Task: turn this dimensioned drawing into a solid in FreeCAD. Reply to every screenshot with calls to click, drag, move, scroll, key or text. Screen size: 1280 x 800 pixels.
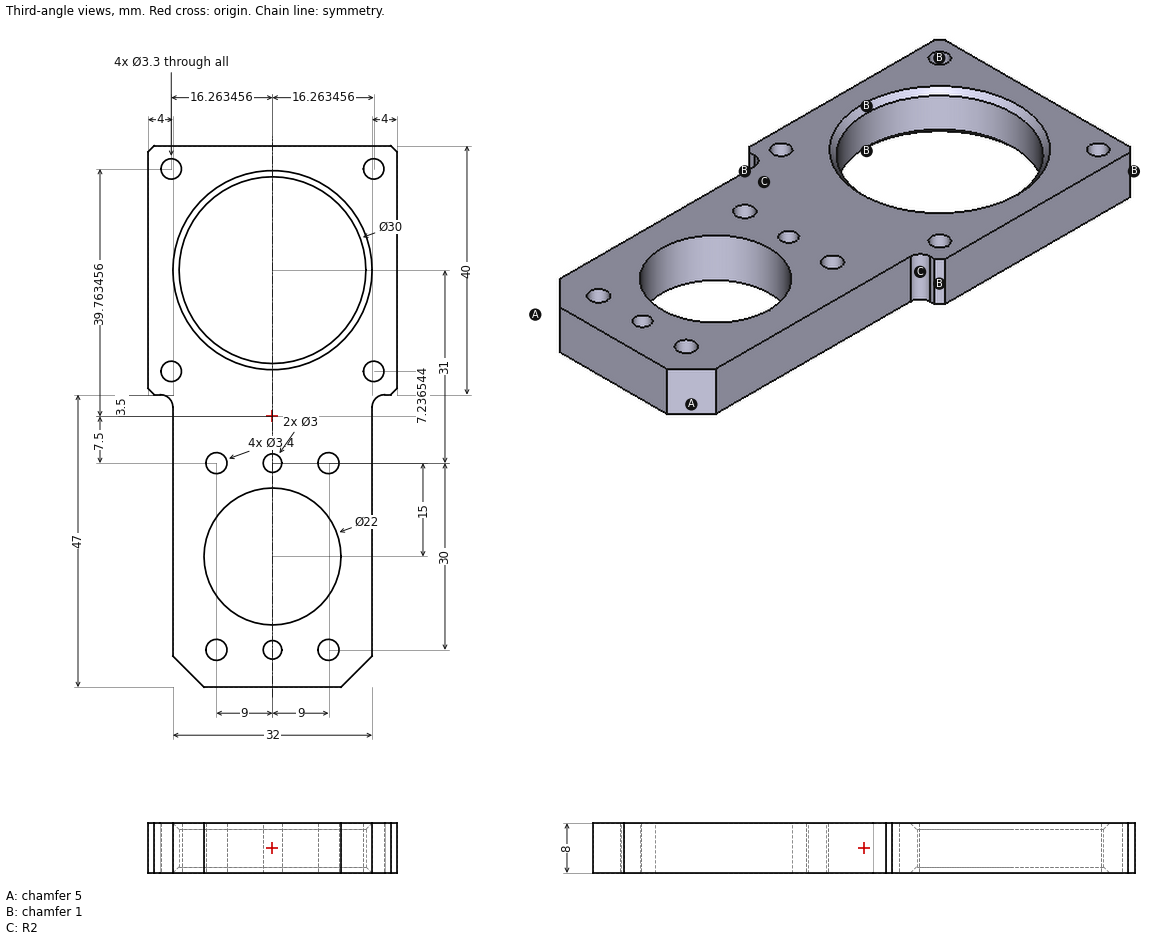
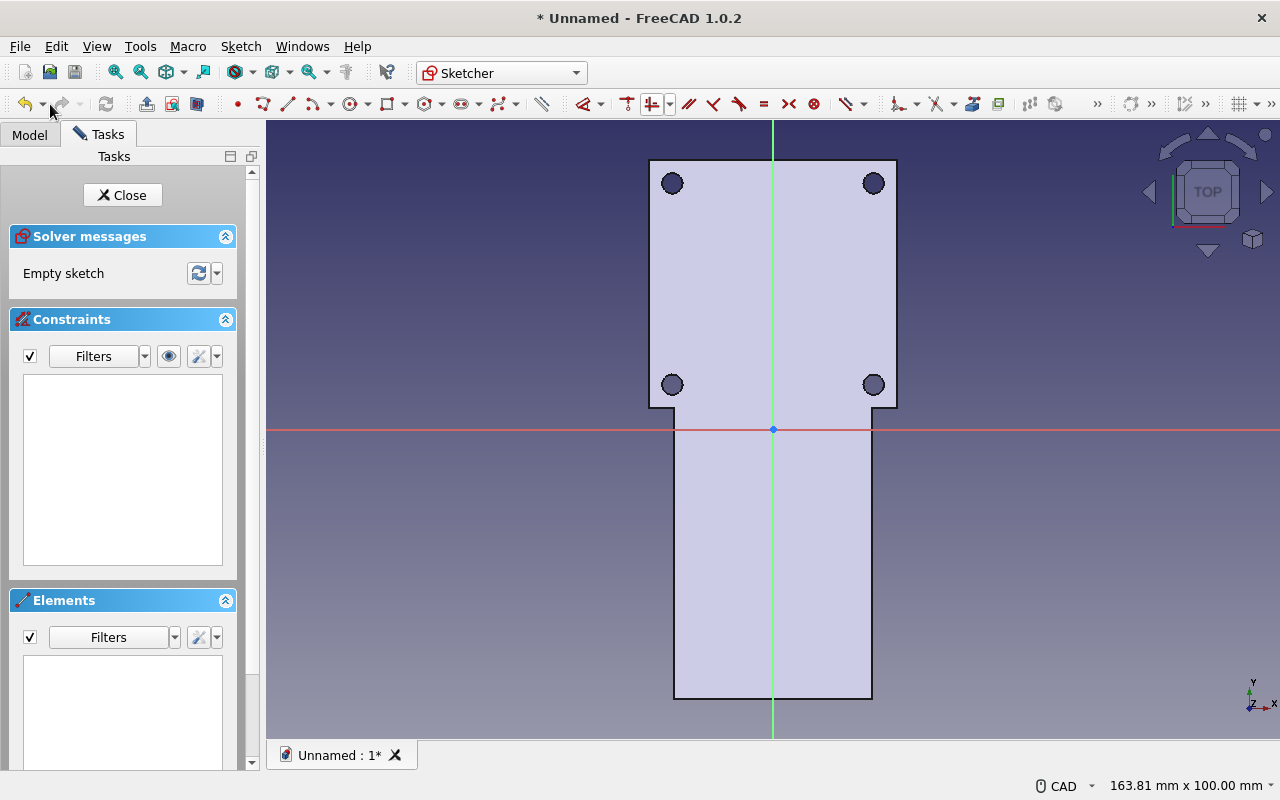
scroll(912, 711, up, 2)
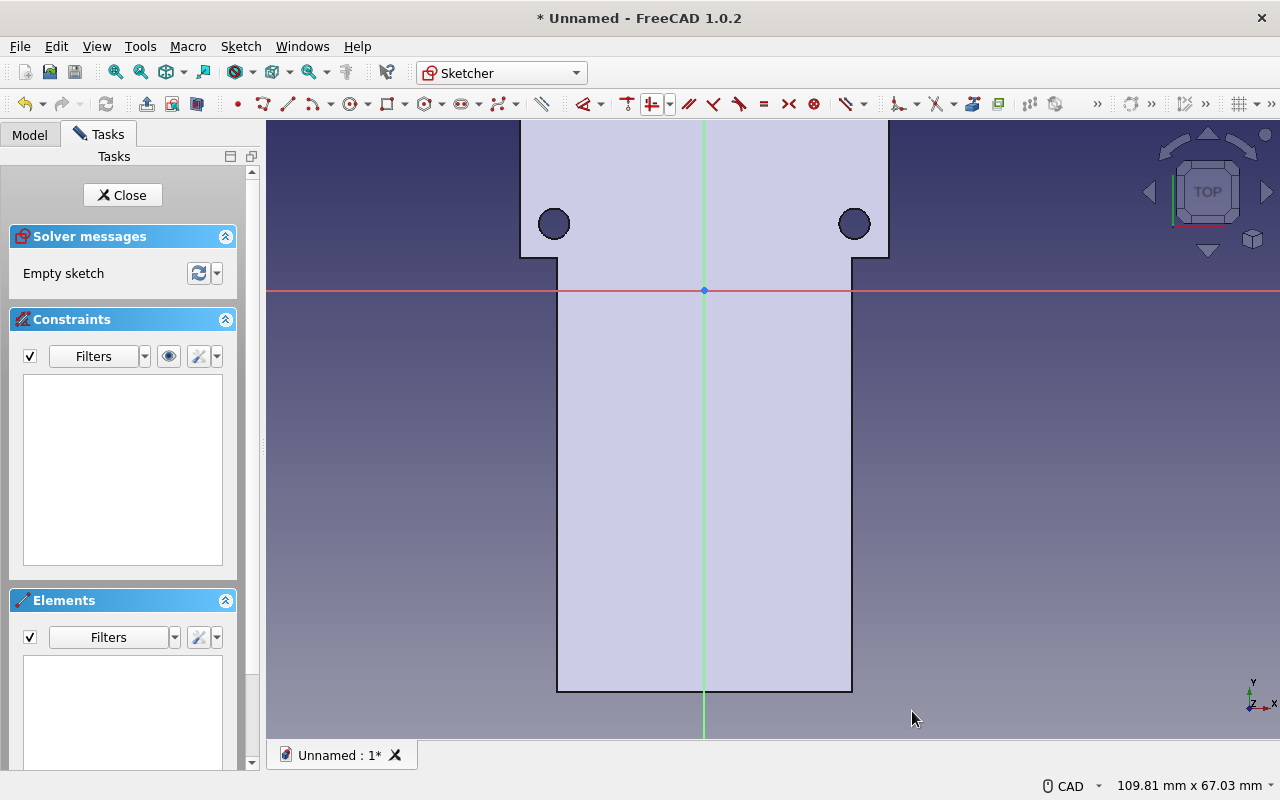
click(350, 104)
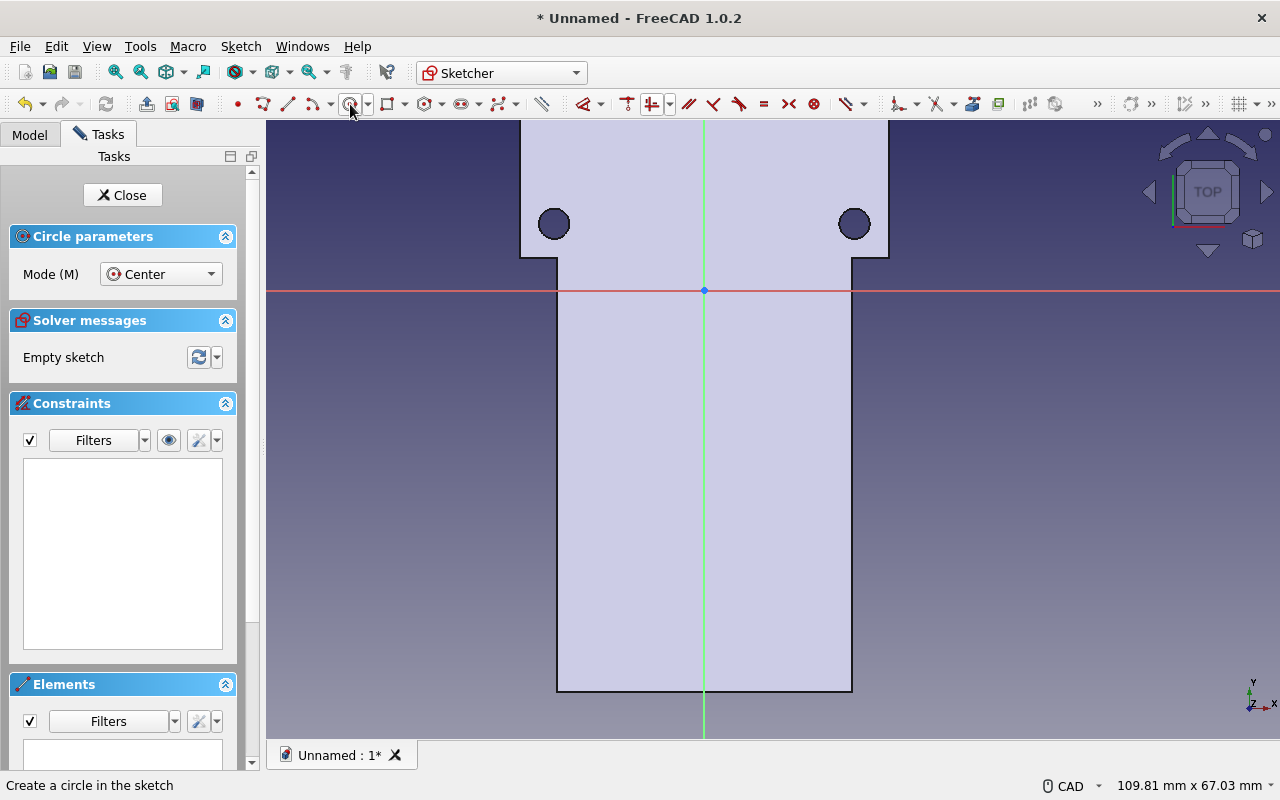
scroll(621, 360, up, 2)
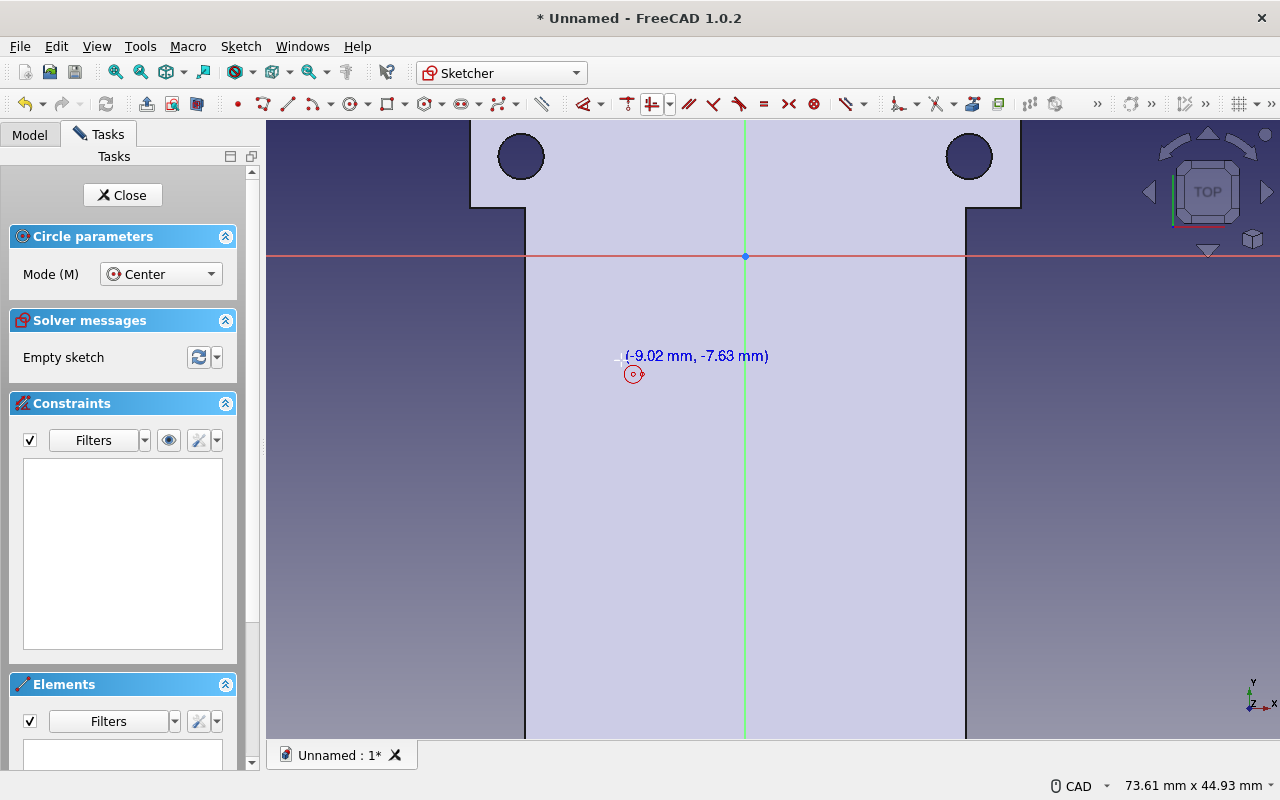
click(621, 360)
click(638, 343)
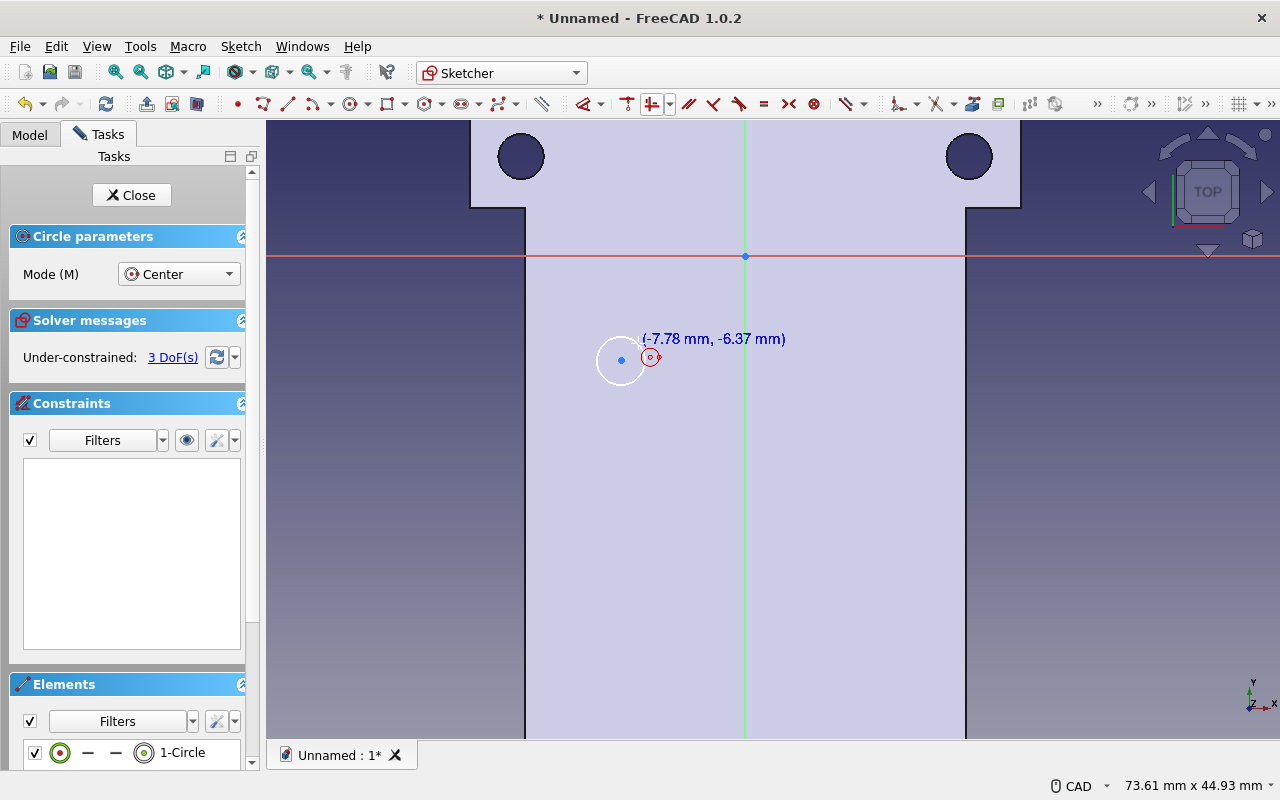
click(869, 360)
click(886, 343)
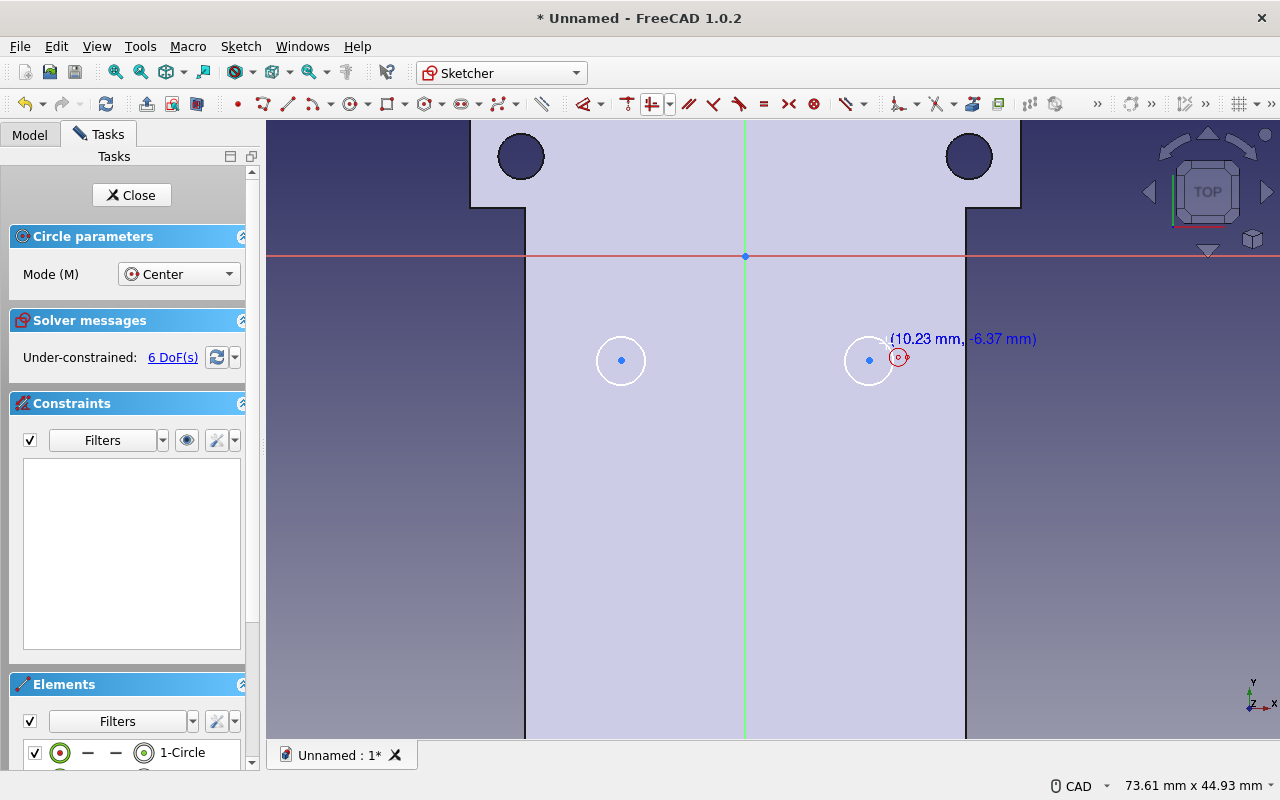
scroll(622, 233, down, 2)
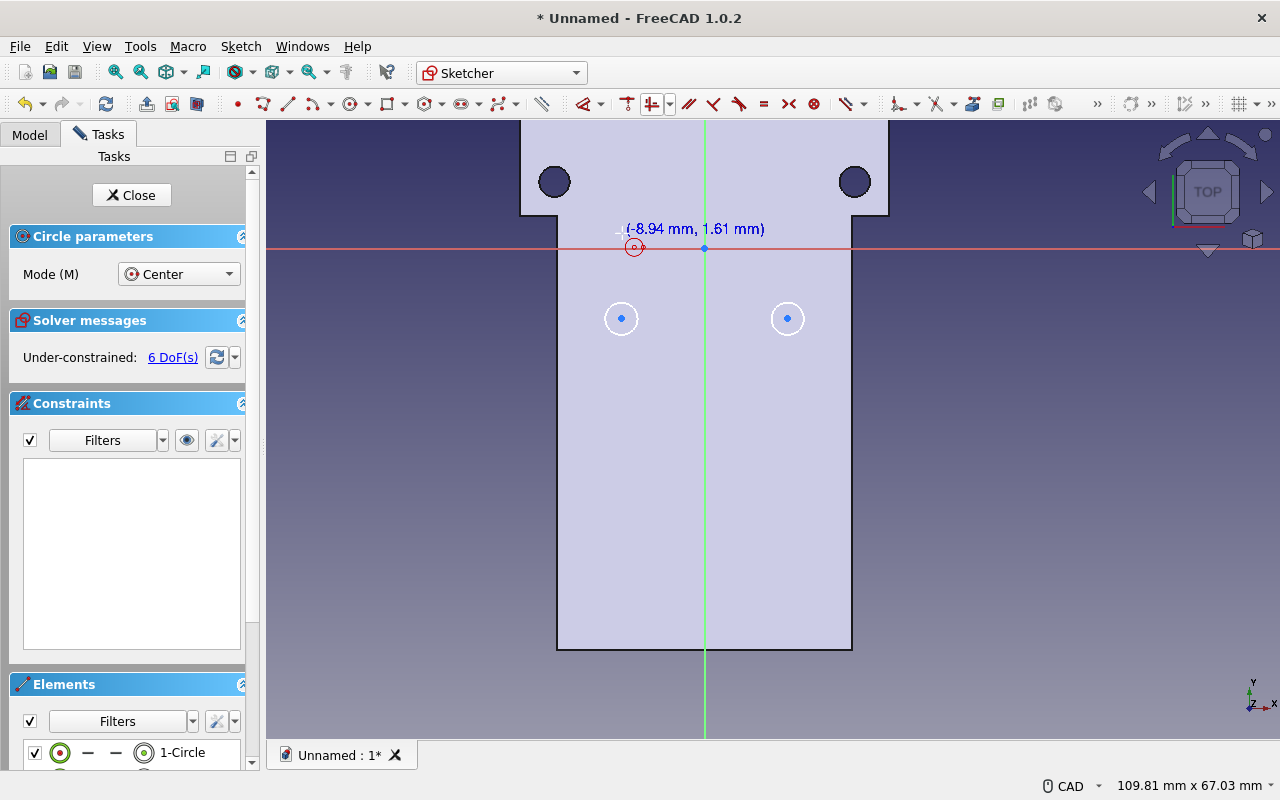
scroll(788, 595, up, 2)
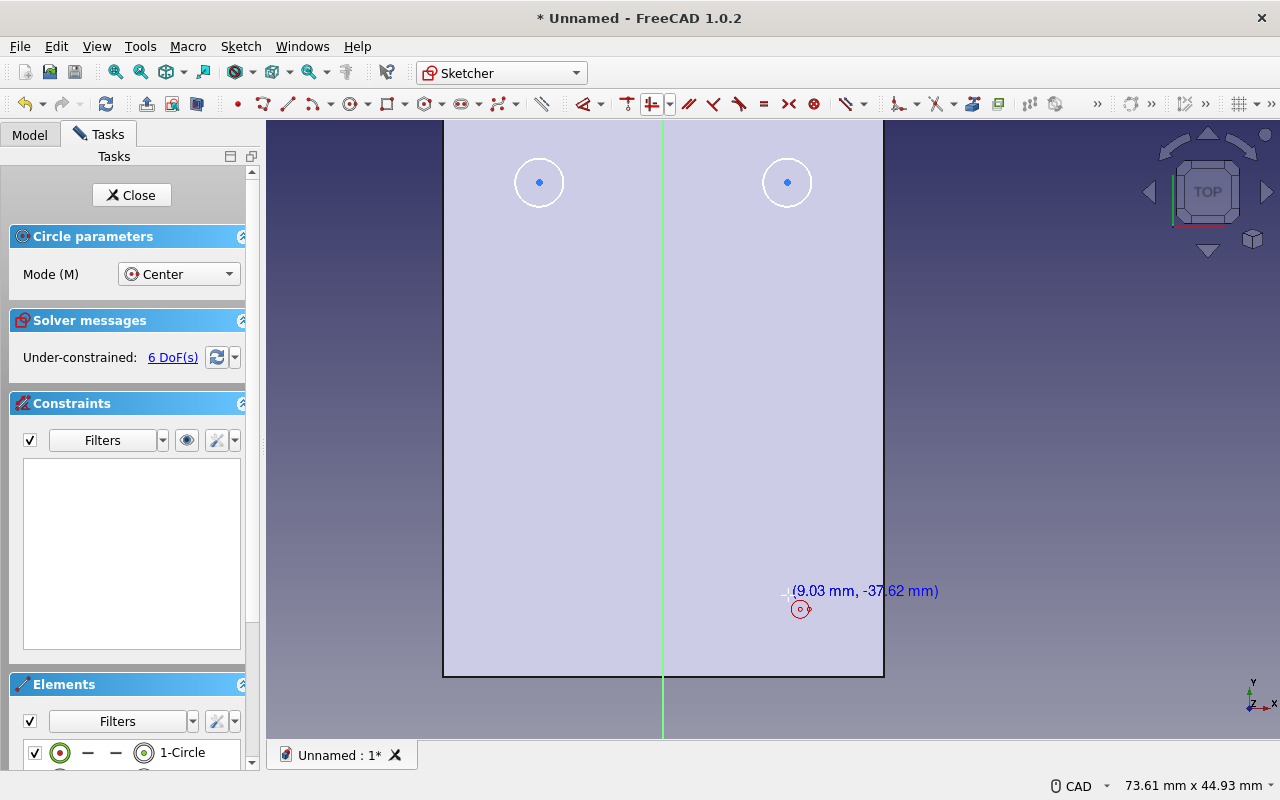
click(787, 595)
click(804, 578)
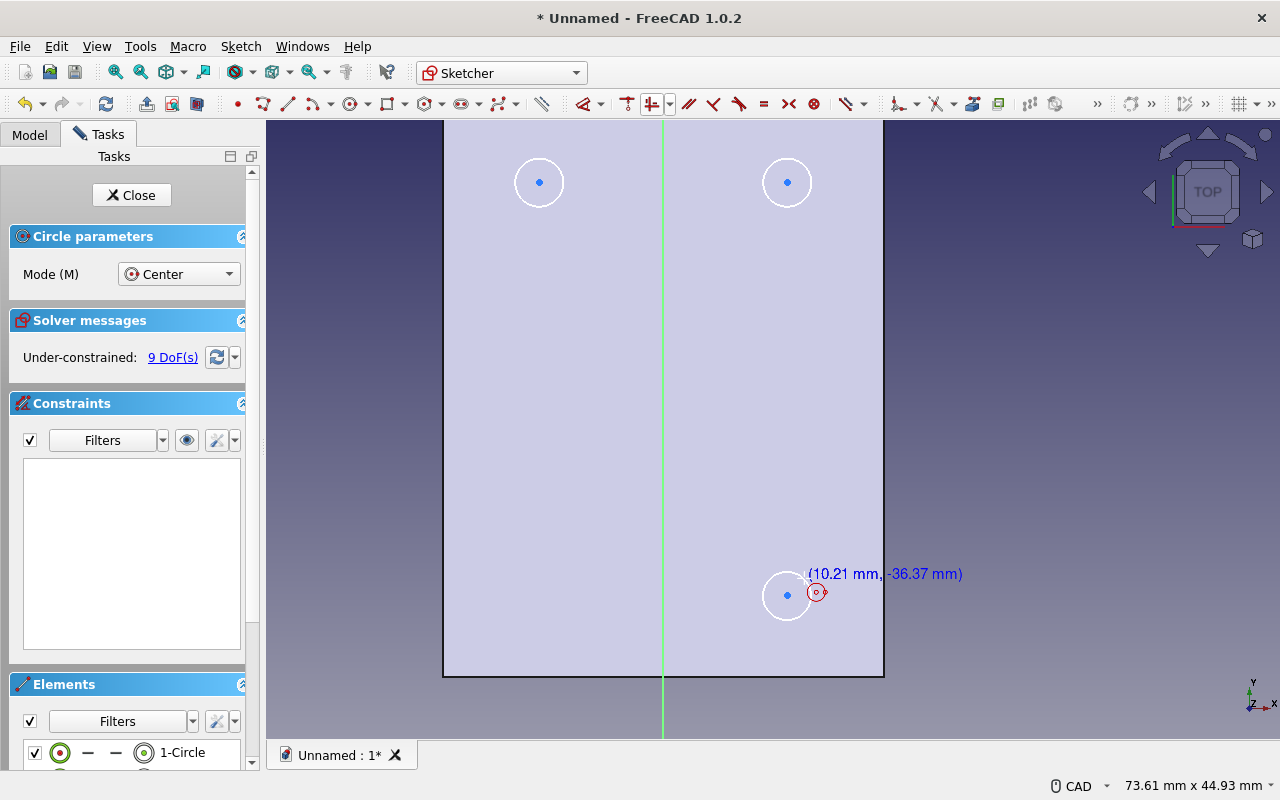
click(539, 595)
click(556, 578)
key(Escape)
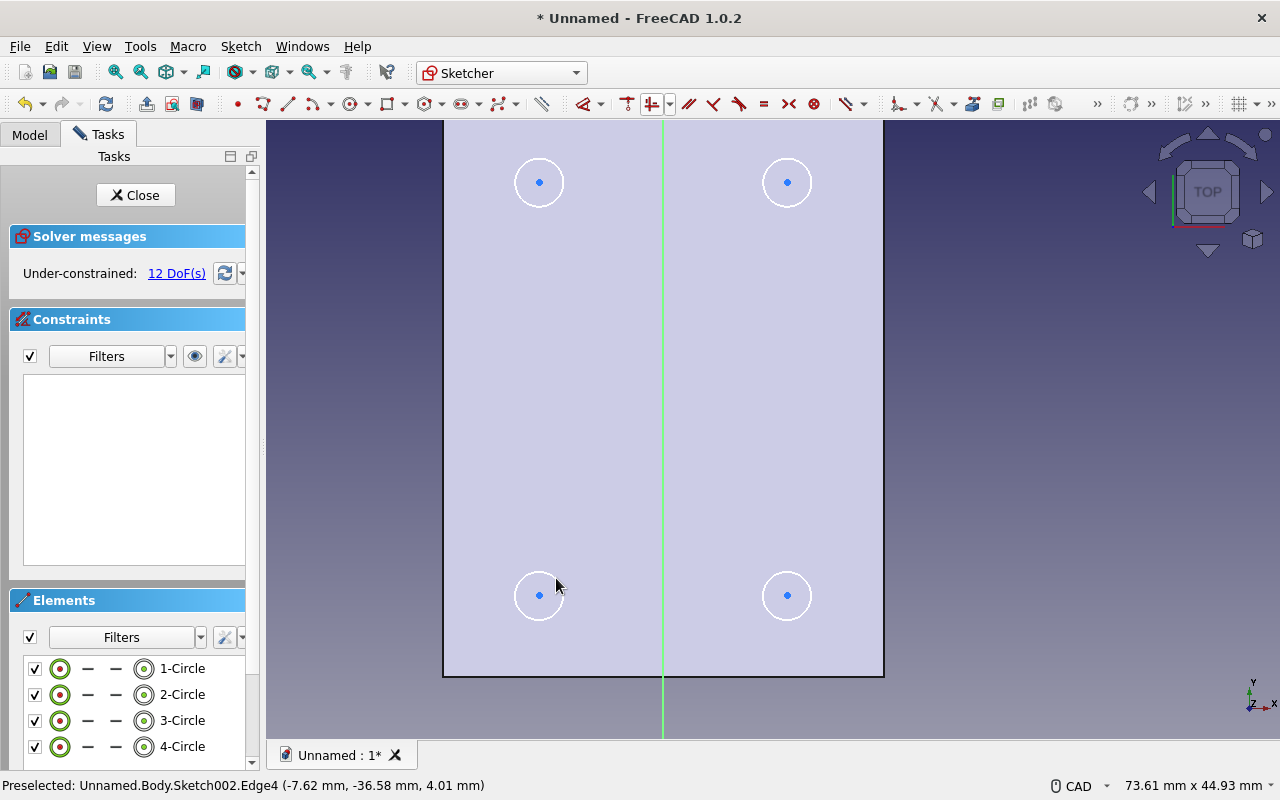
click(556, 166)